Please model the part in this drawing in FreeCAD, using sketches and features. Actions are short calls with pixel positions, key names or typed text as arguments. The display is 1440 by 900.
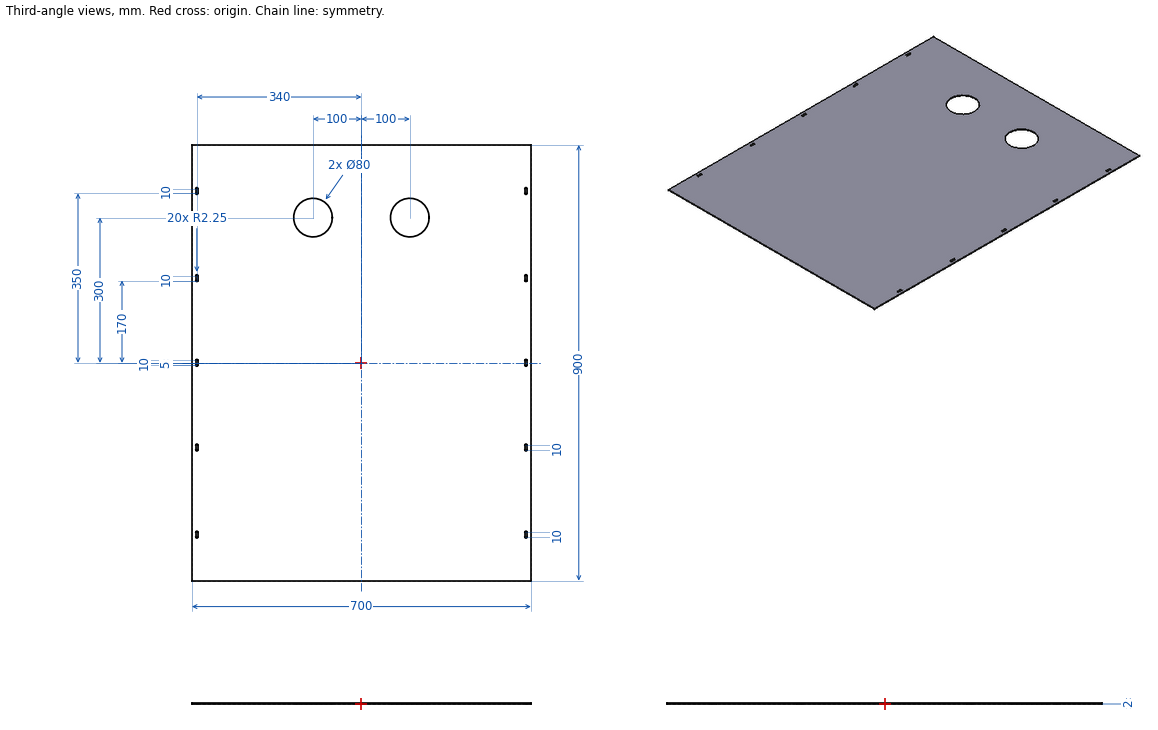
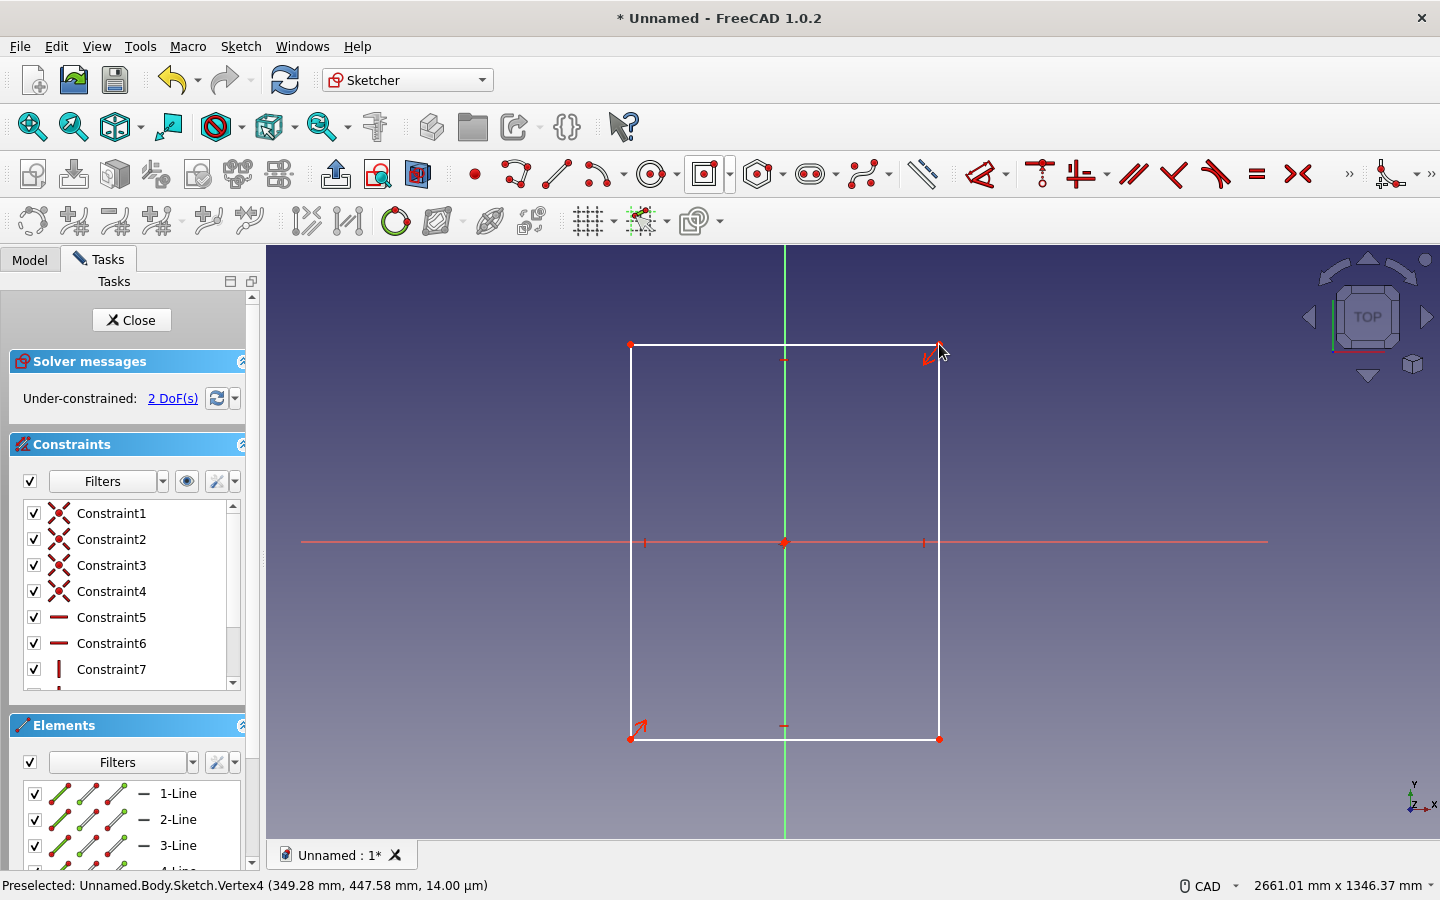
key(d)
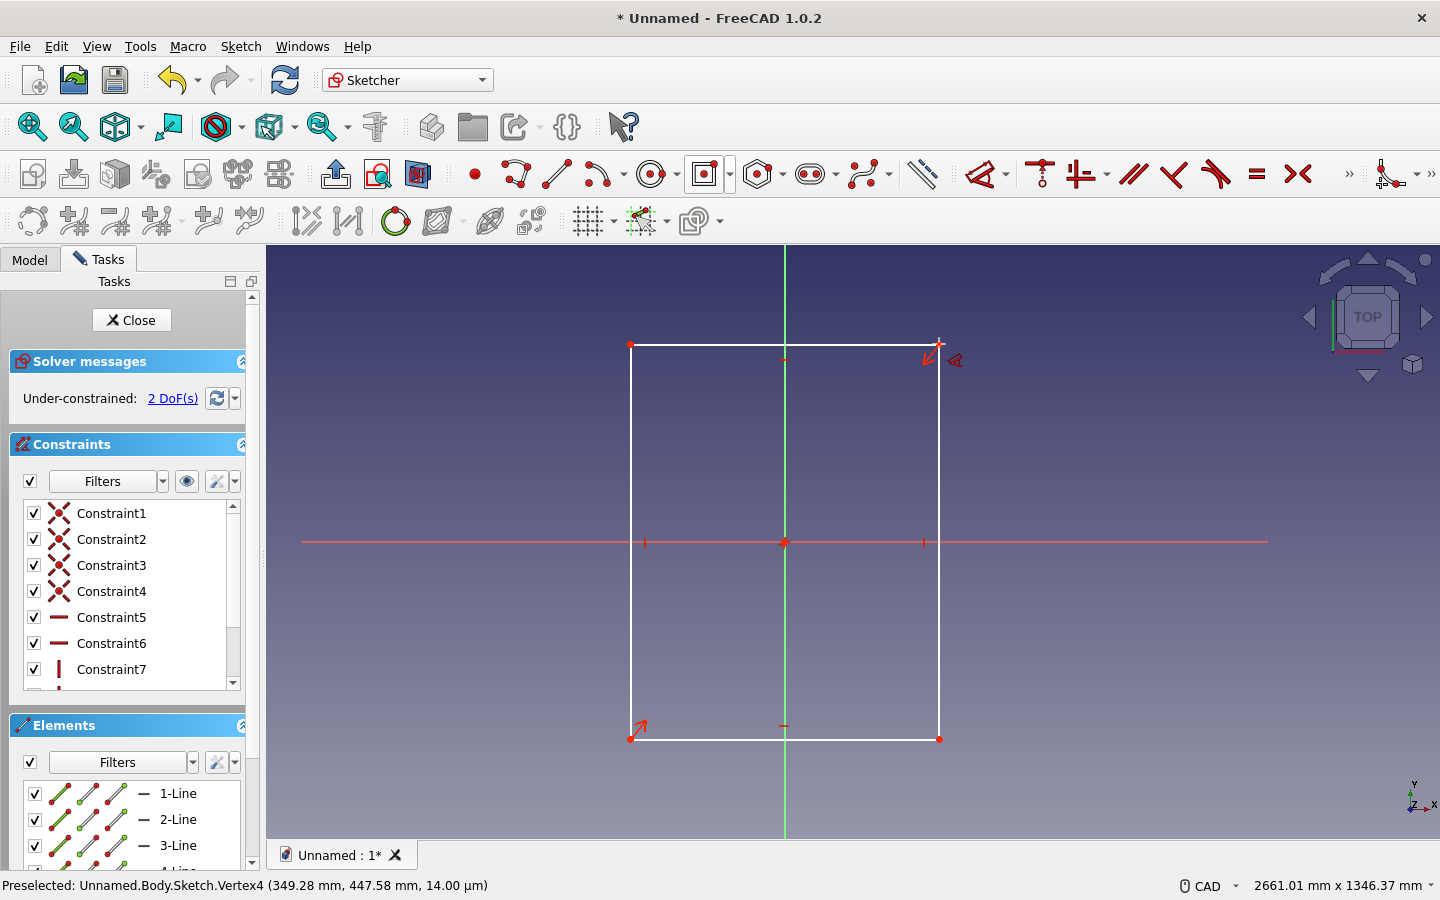
click(723, 740)
click(714, 774)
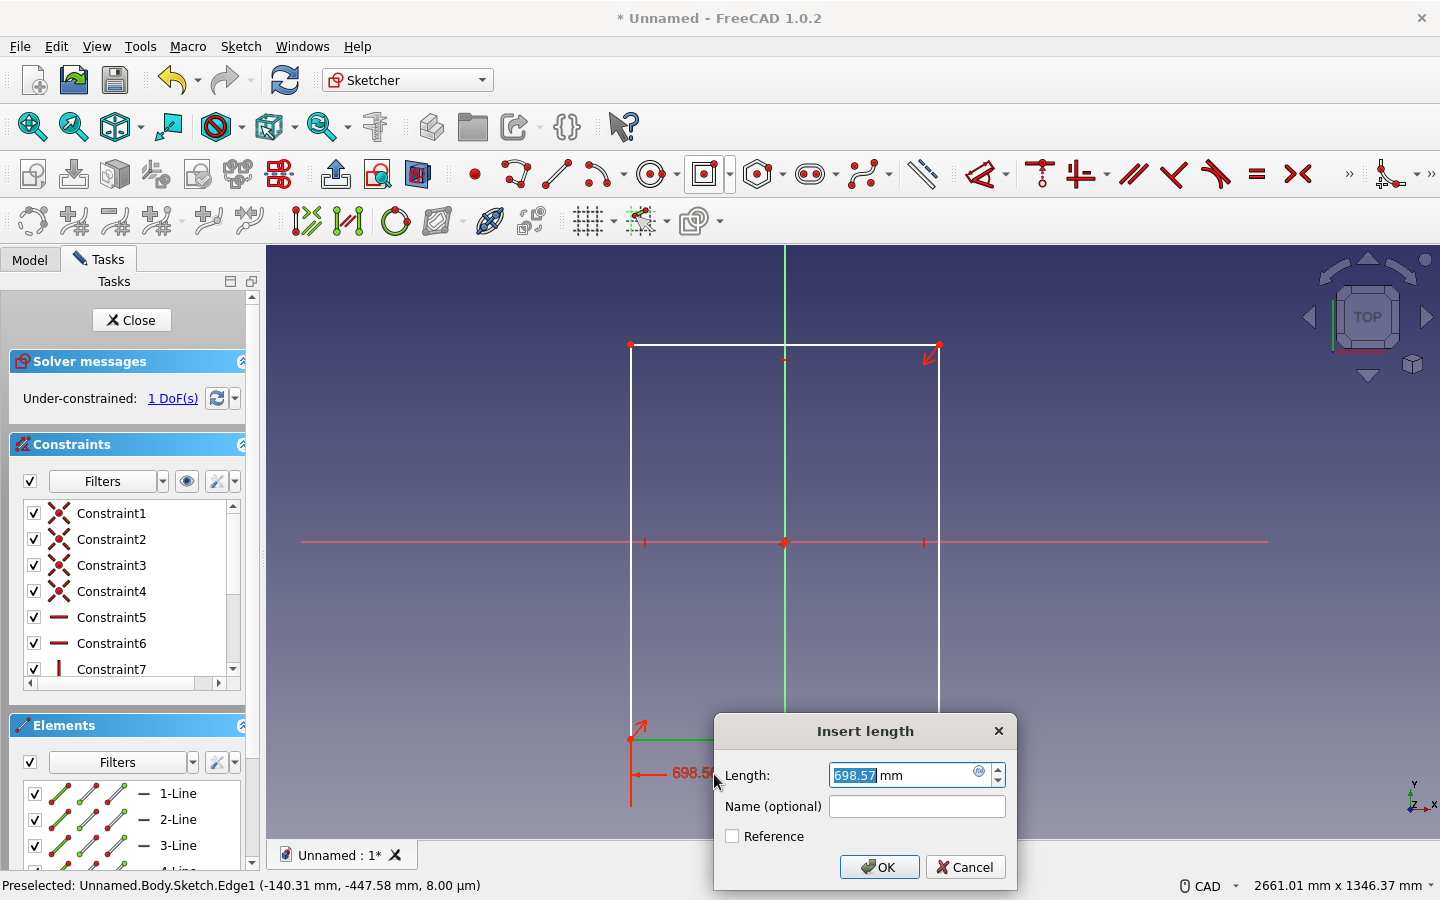
text(700)
key(Return)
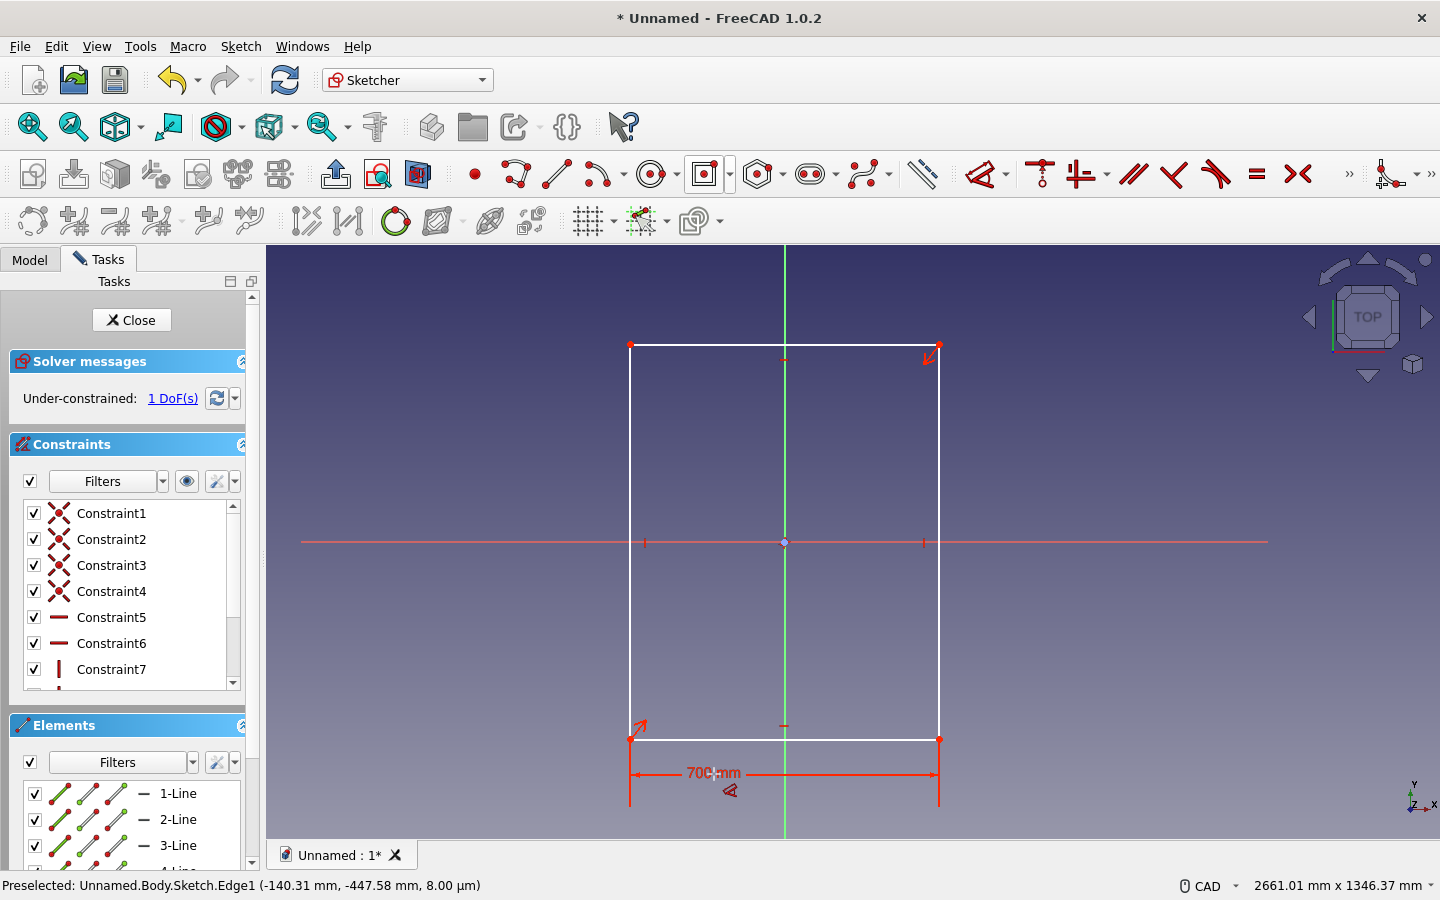
click(939, 621)
click(973, 452)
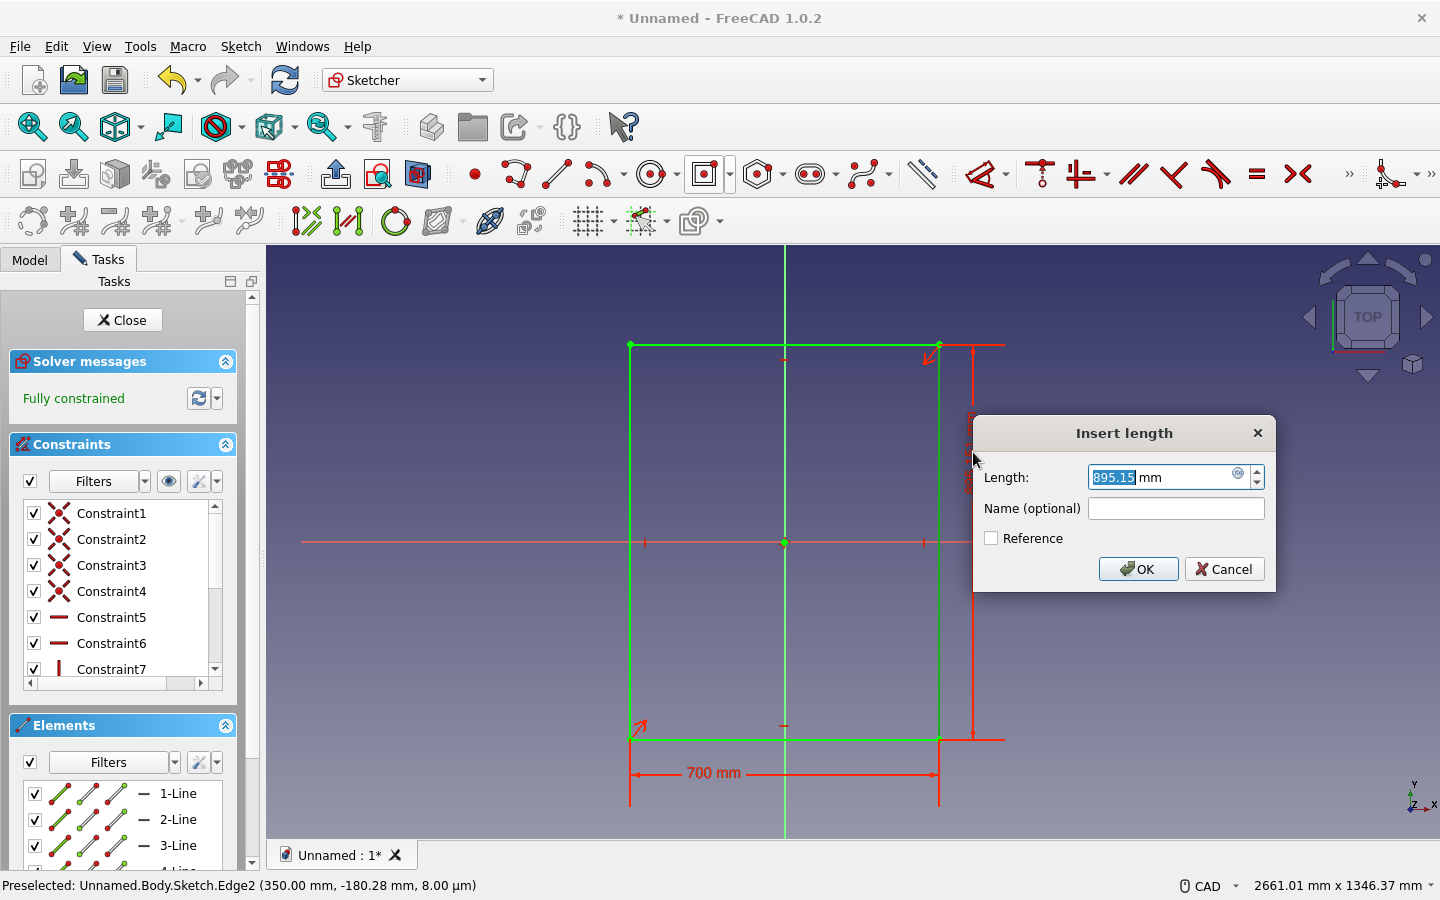
text(900)
key(Return)
key(Escape)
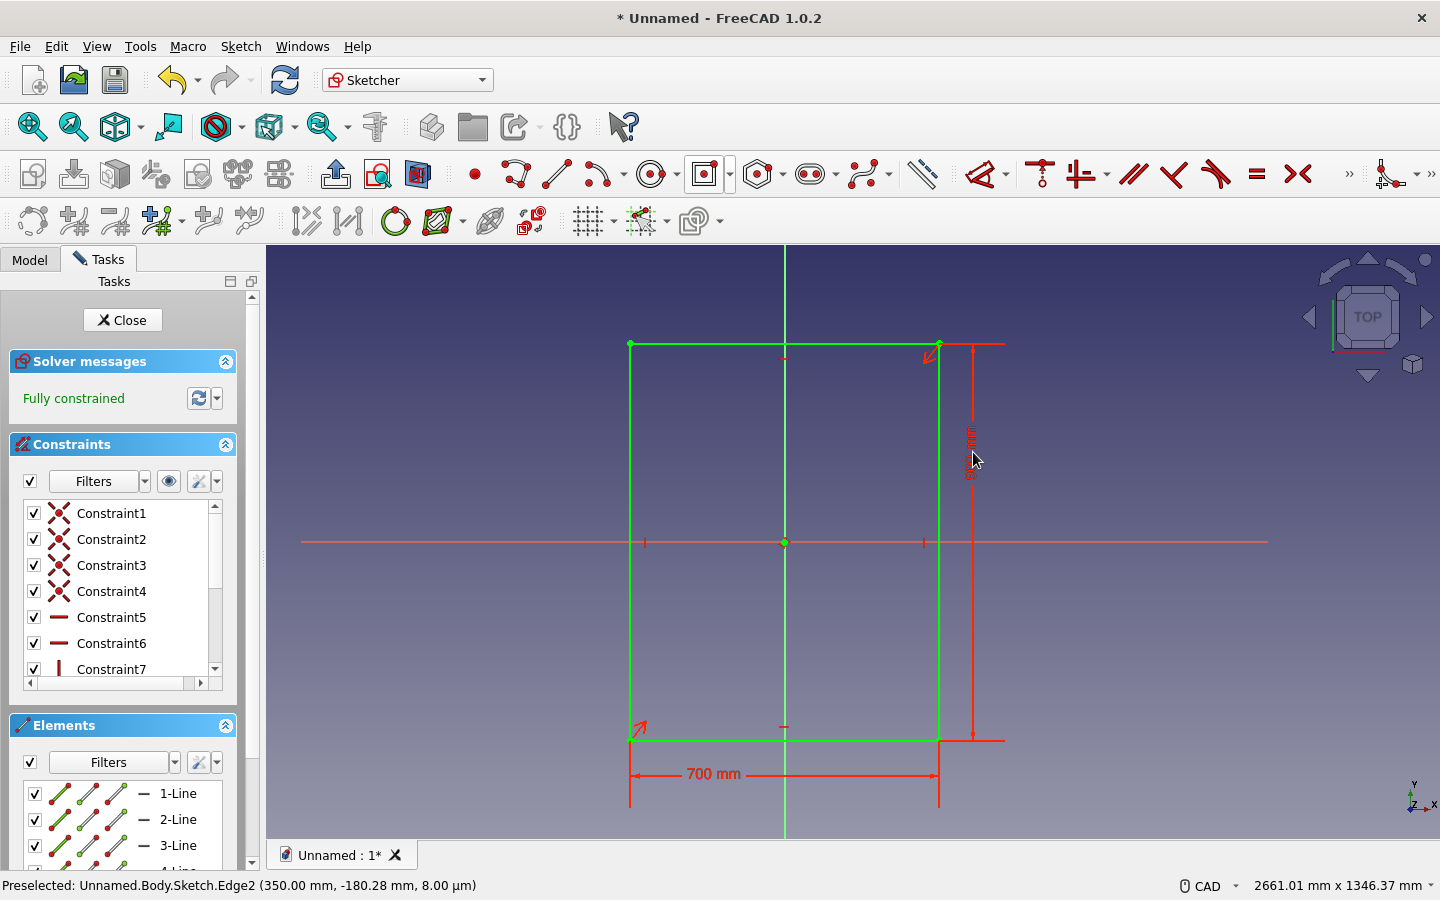
click(123, 320)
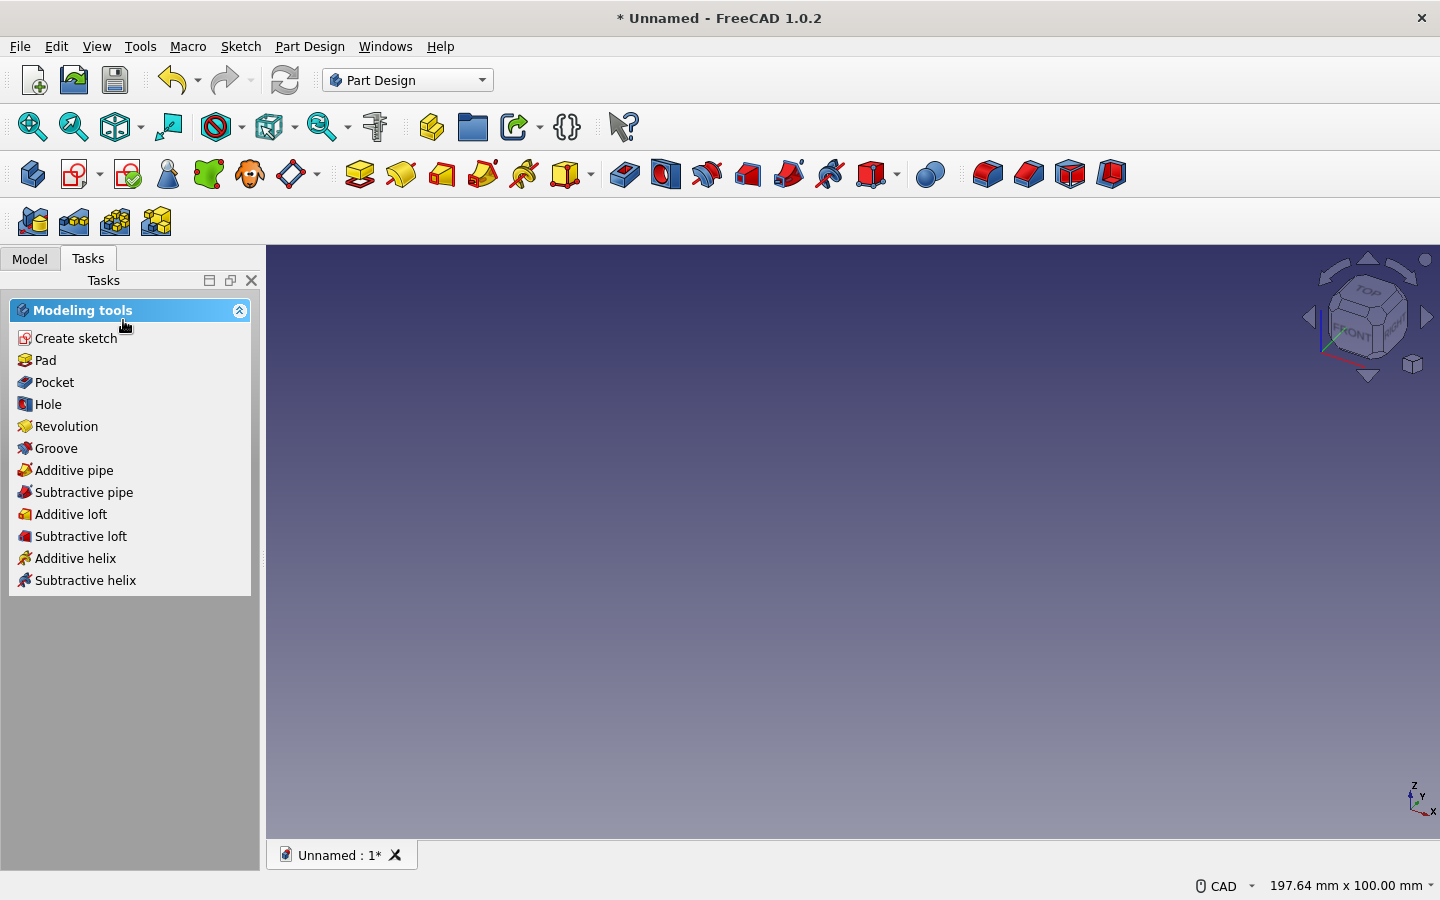
click(360, 174)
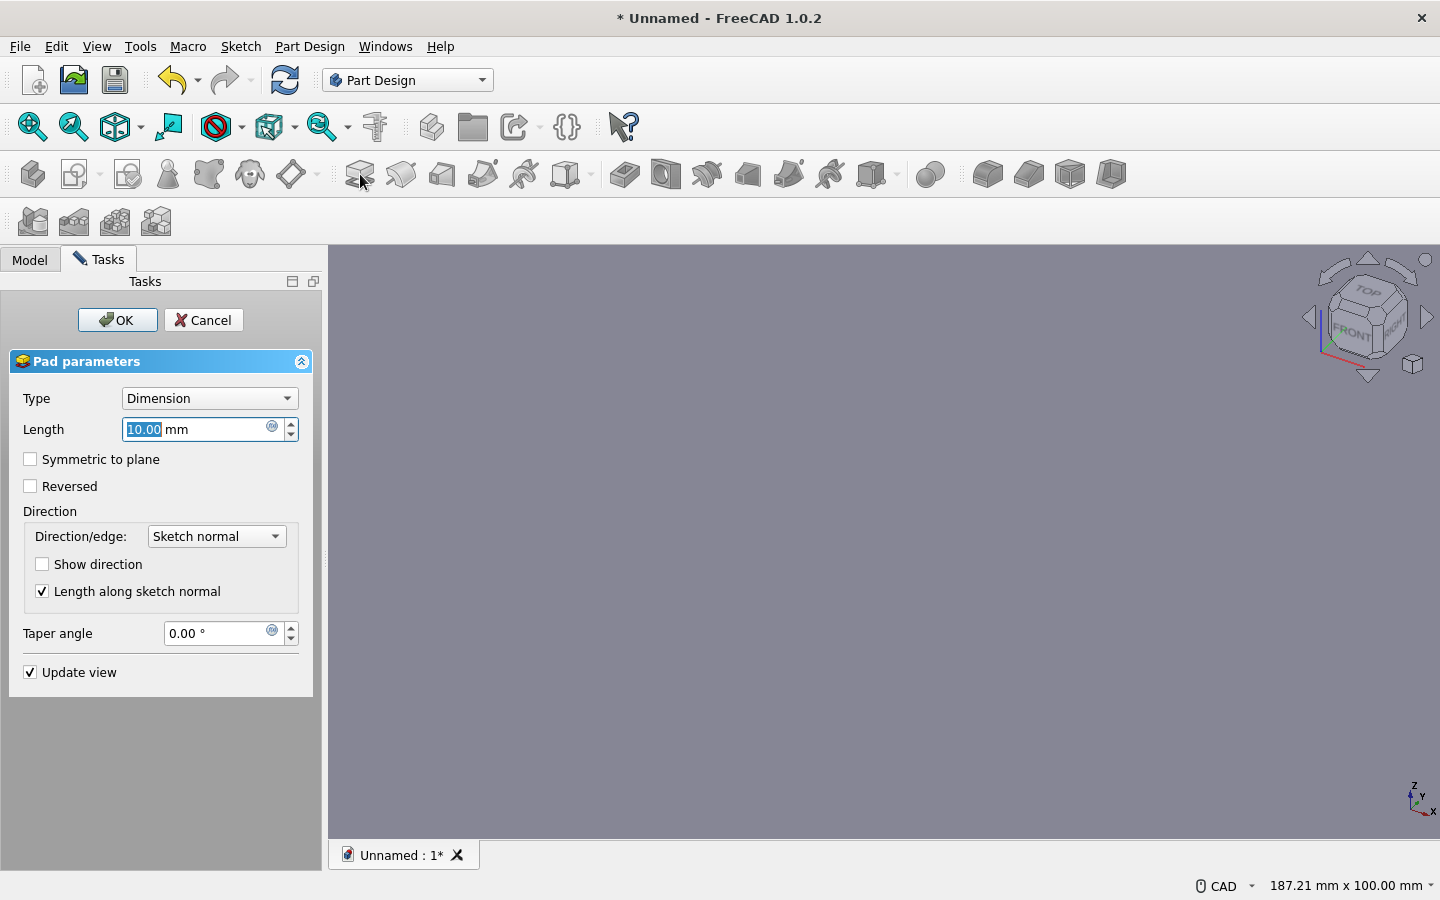
text(2)
key(Tab)